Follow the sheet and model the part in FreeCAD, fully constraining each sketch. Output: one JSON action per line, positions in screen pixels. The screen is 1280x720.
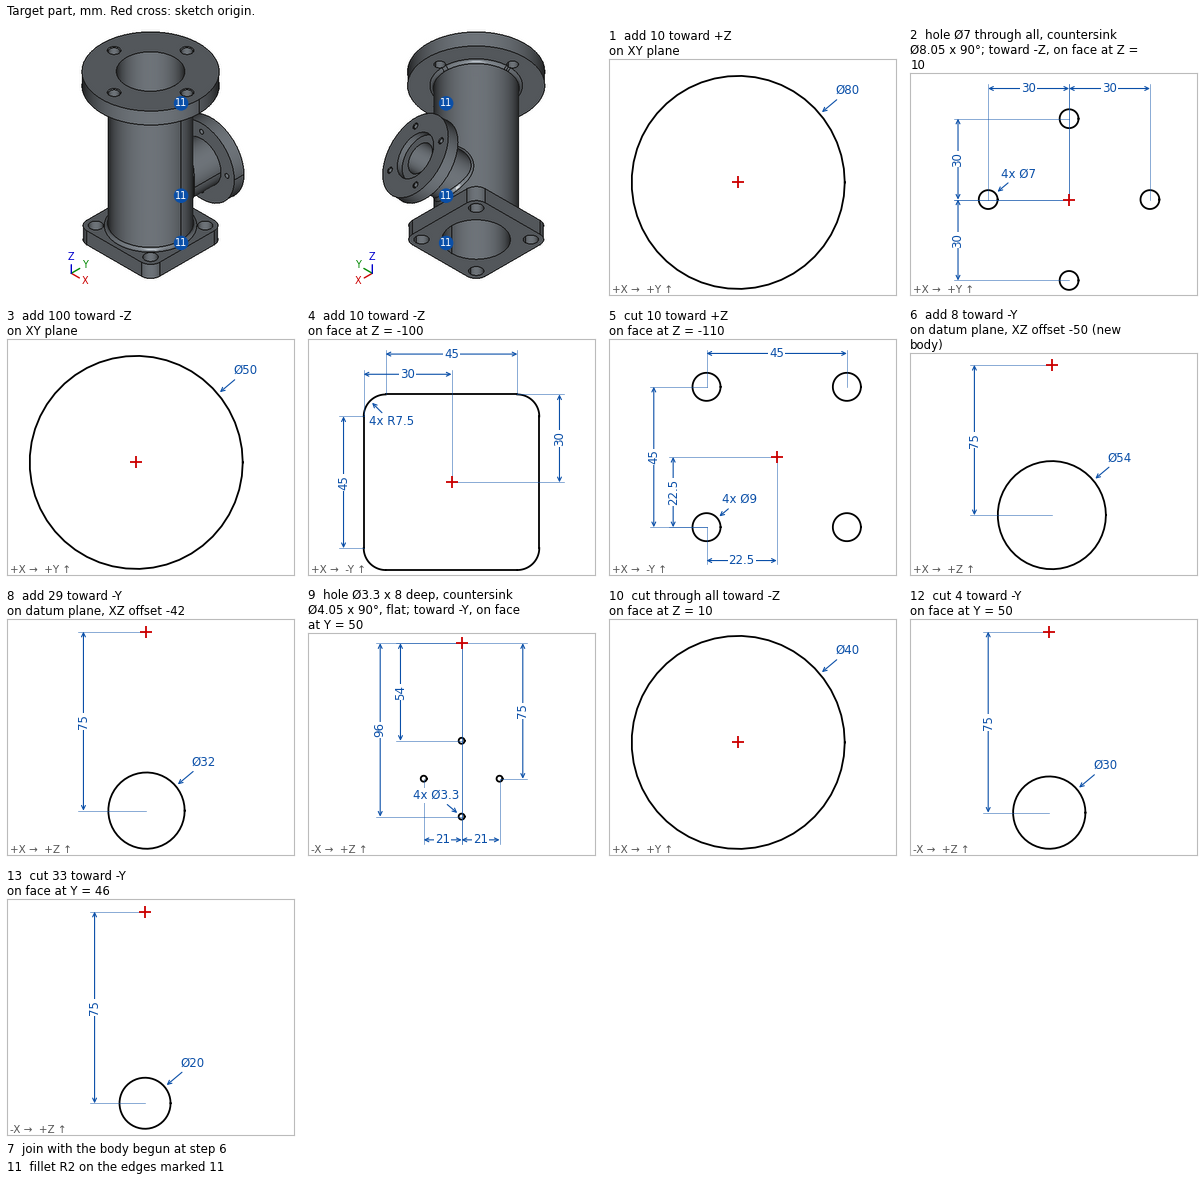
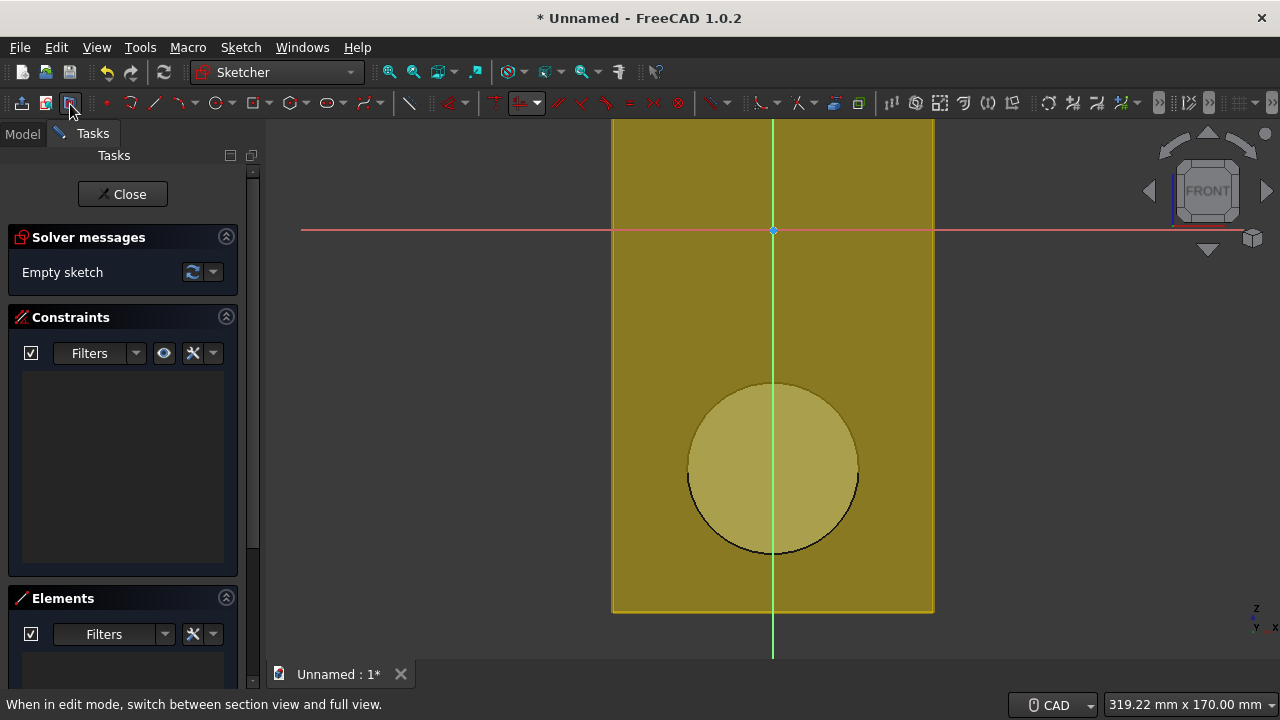
{"action": "scroll", "coordinate": [803, 503], "scroll_direction": "up", "scroll_amount": 6}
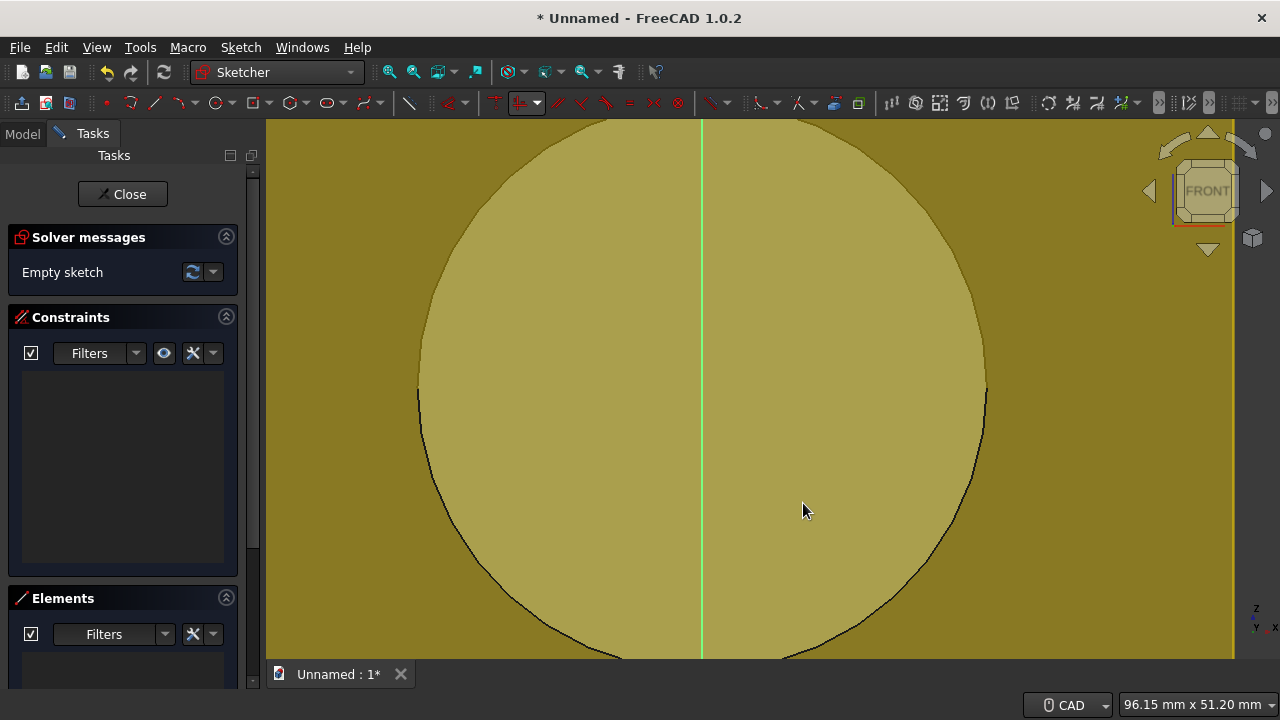
{"action": "left_click", "coordinate": [216, 104]}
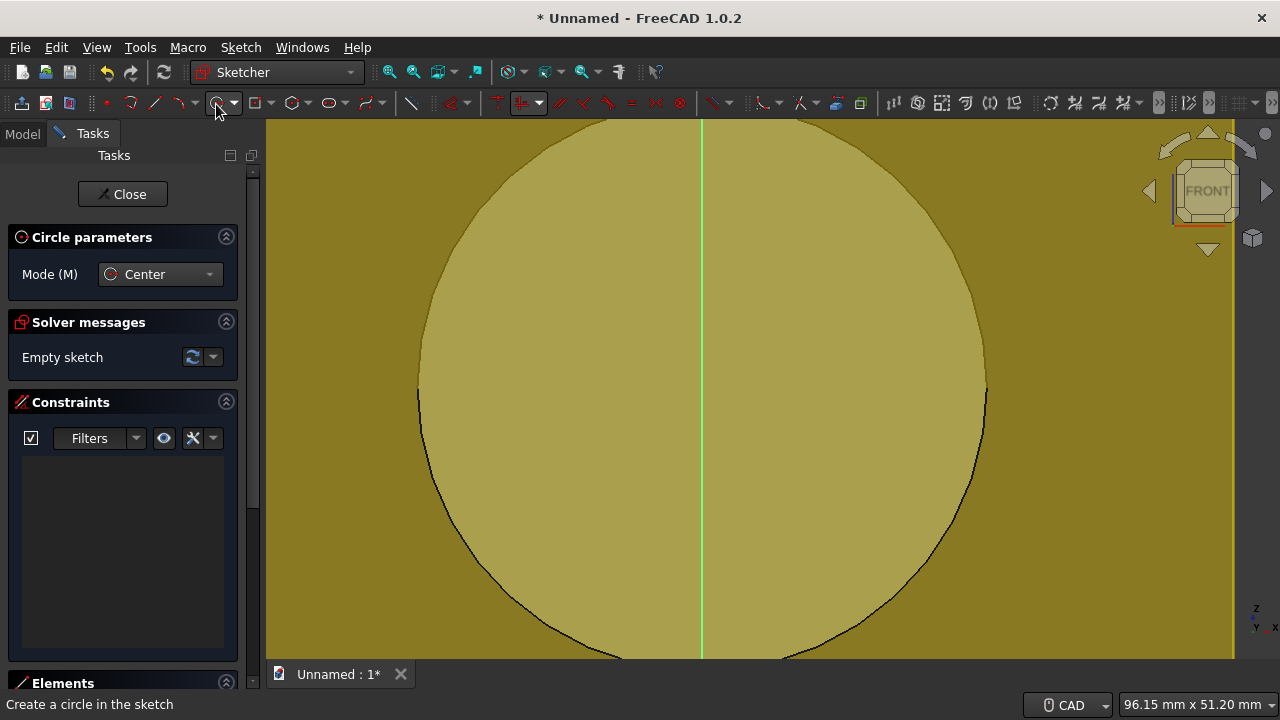
{"action": "left_click", "coordinate": [702, 387]}
{"action": "mouse_move", "coordinate": [821, 267]}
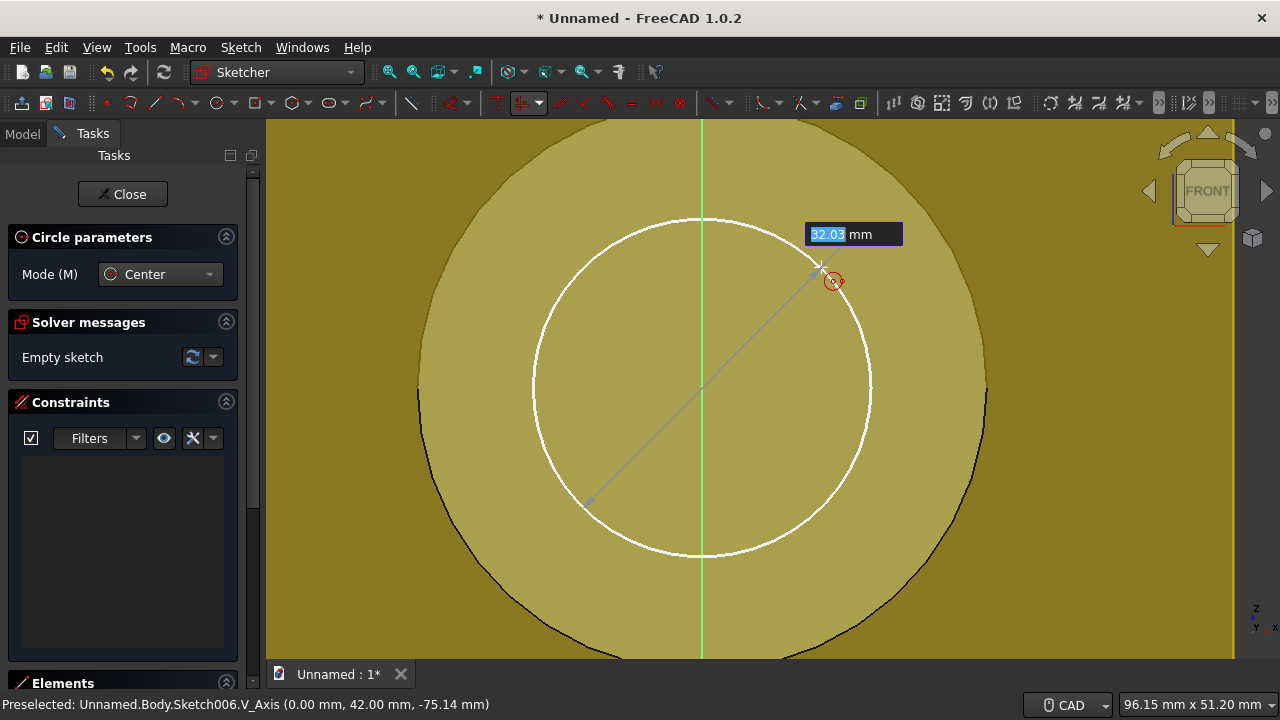
{"action": "type", "text": "32"}
{"action": "key", "text": "Return"}
{"action": "key", "text": "Escape"}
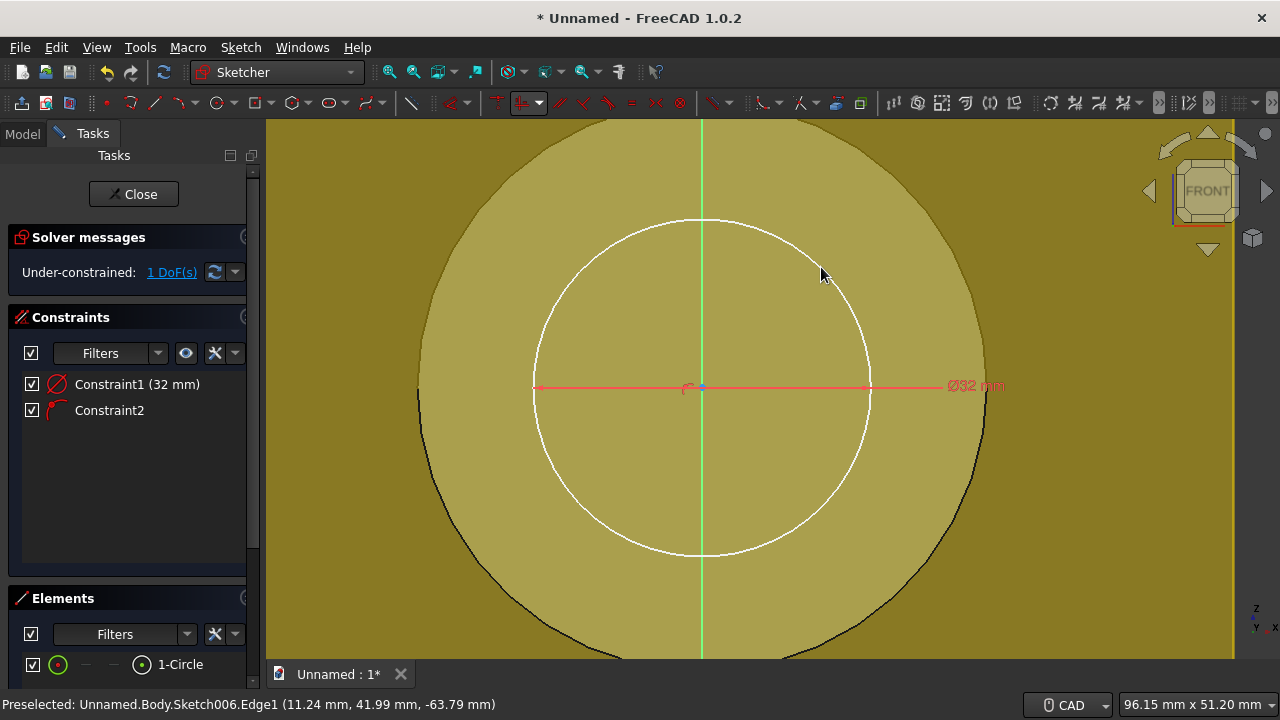
{"action": "left_click", "coordinate": [450, 104]}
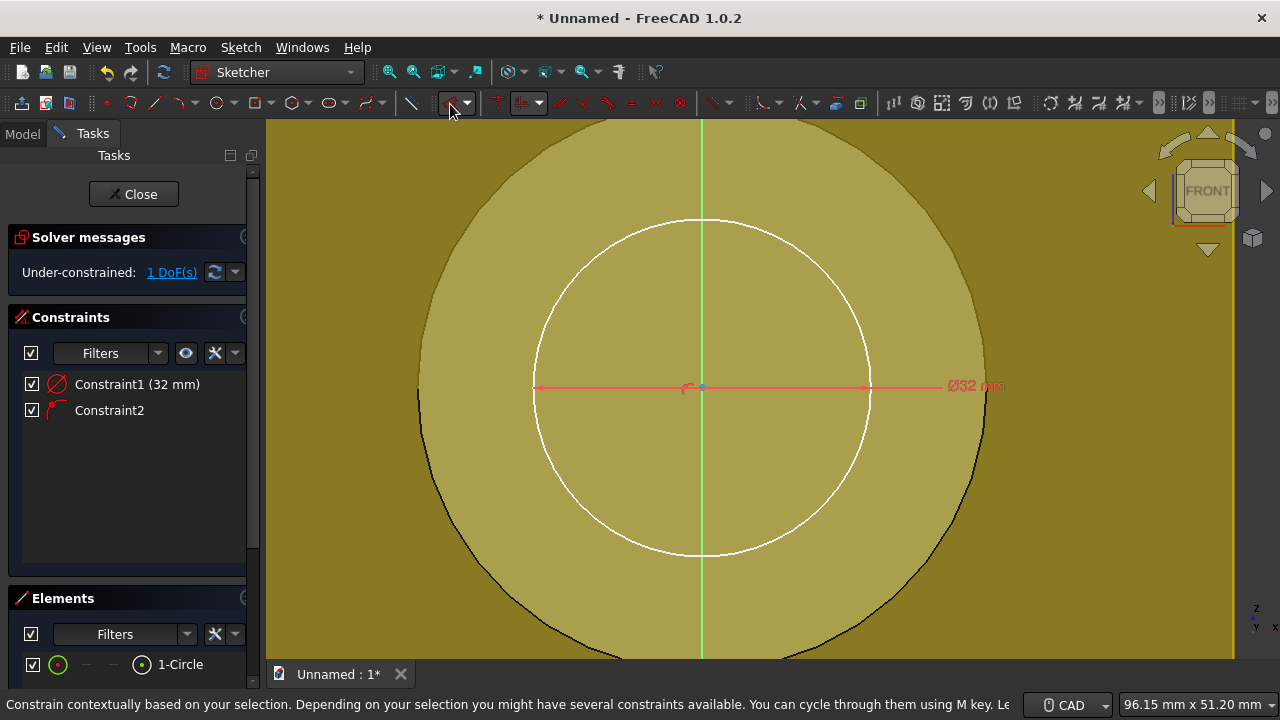
{"action": "left_click", "coordinate": [702, 388]}
{"action": "left_click", "coordinate": [736, 268]}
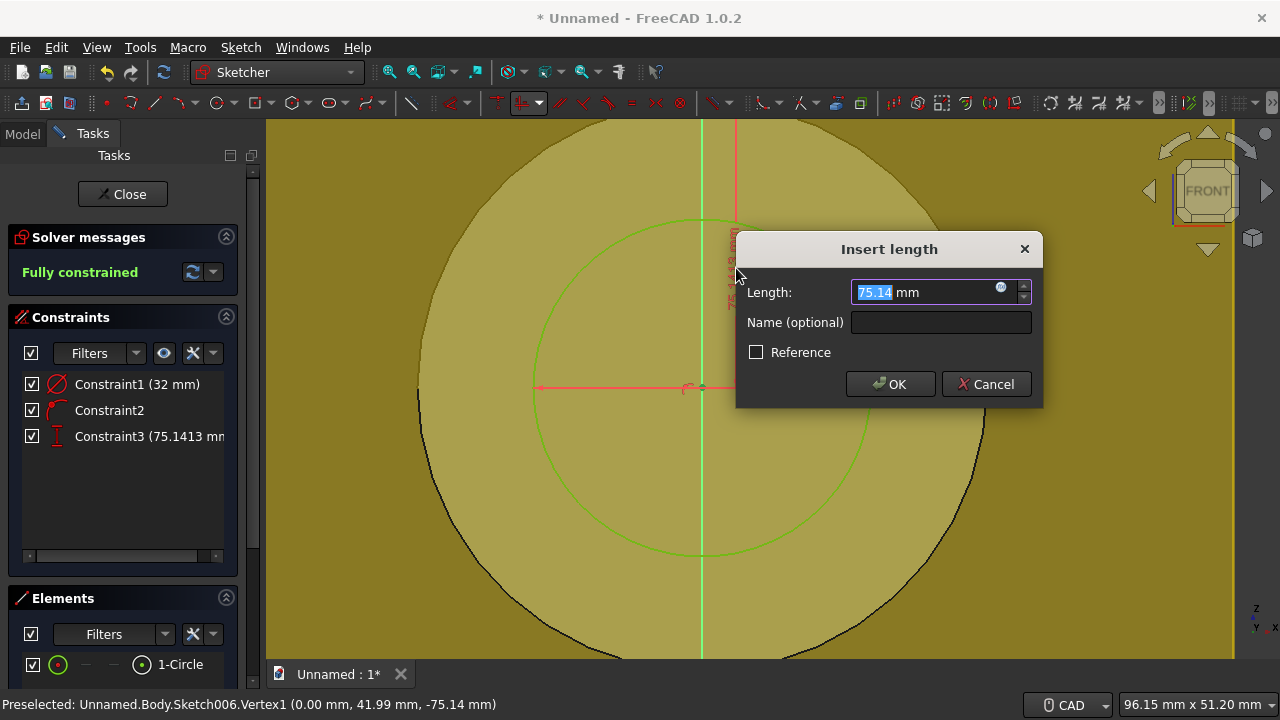
{"action": "type", "text": "75"}
{"action": "key", "text": "Return"}
{"action": "key", "text": "Escape"}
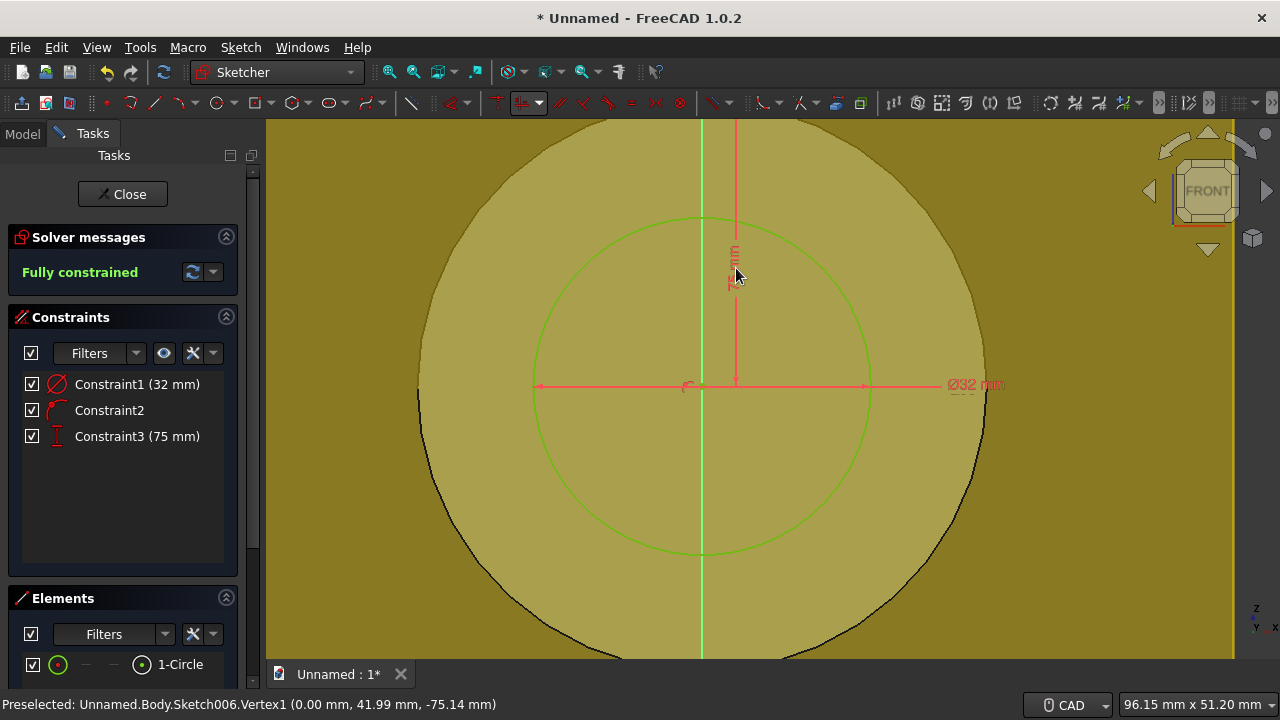
{"action": "left_click", "coordinate": [123, 194]}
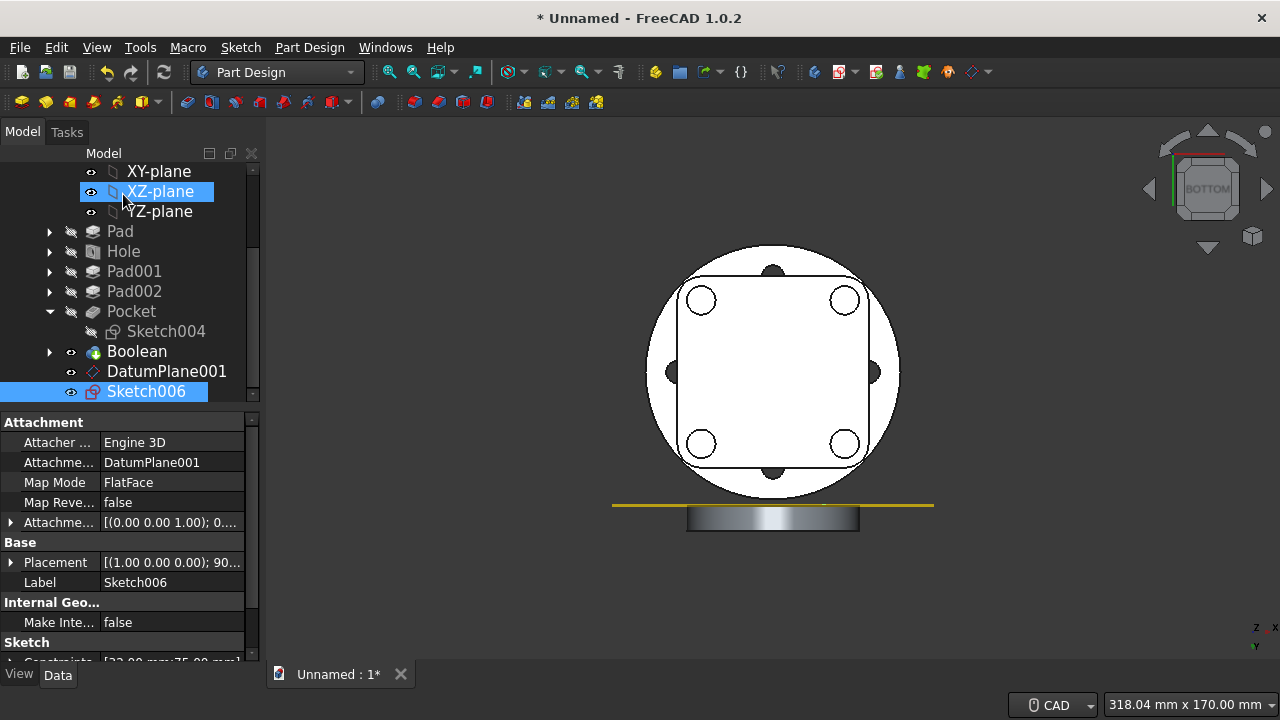
{"action": "left_click", "coordinate": [22, 102]}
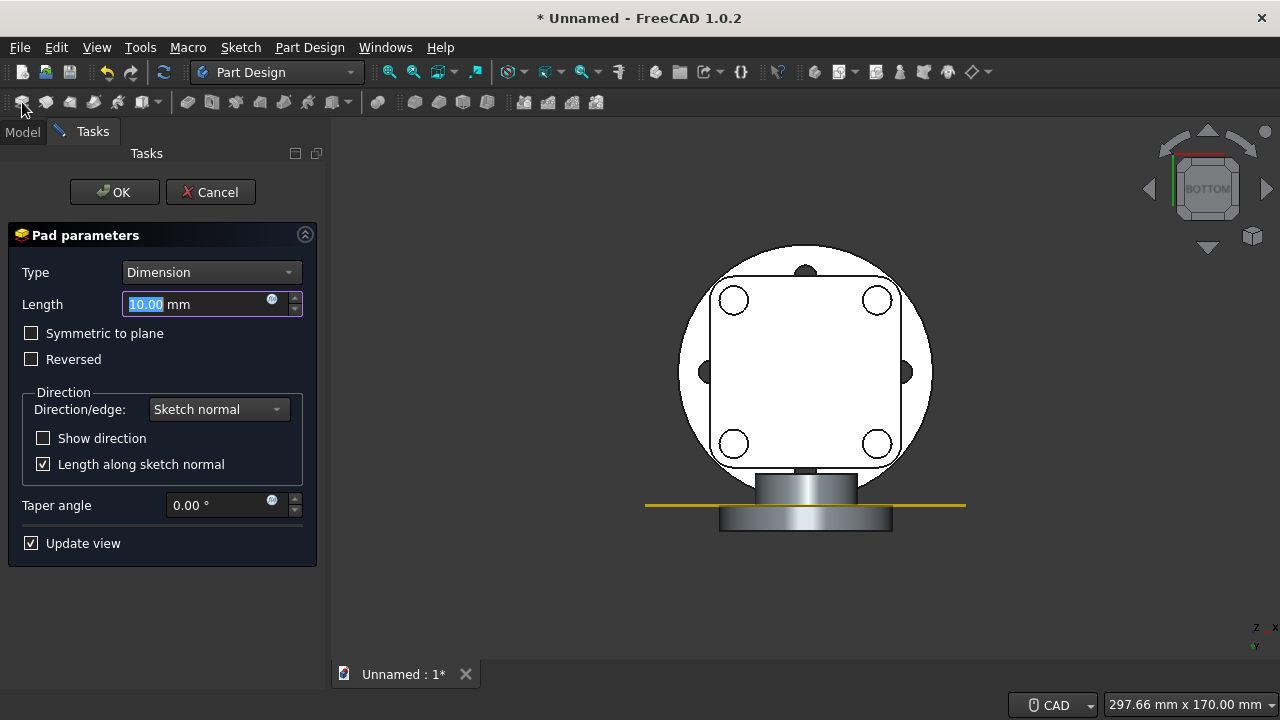
{"action": "type", "text": "29"}
{"action": "key", "text": "Tab"}